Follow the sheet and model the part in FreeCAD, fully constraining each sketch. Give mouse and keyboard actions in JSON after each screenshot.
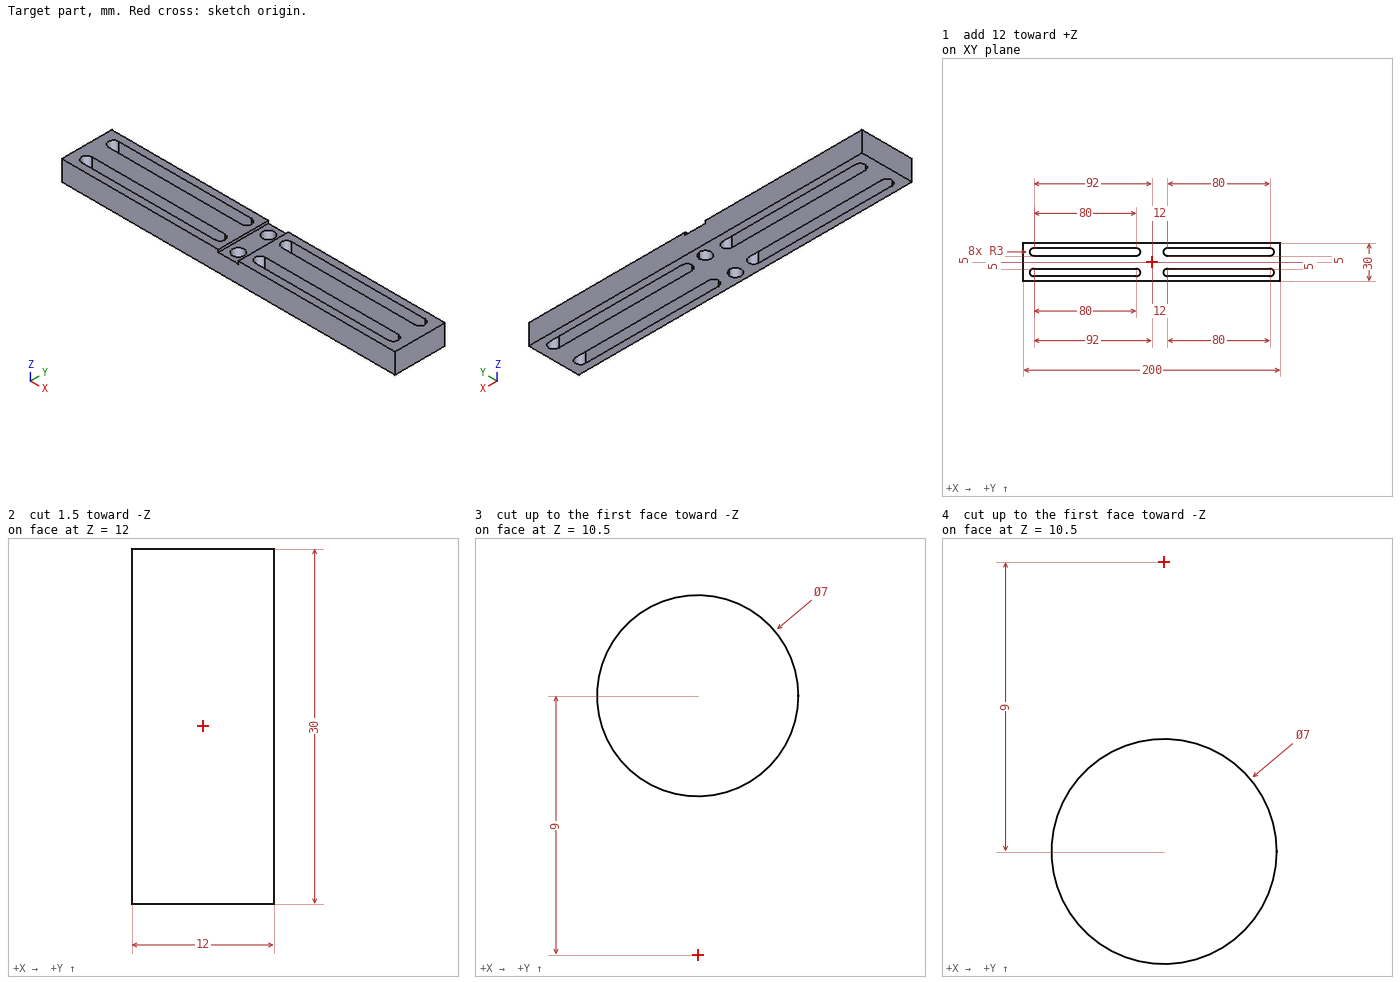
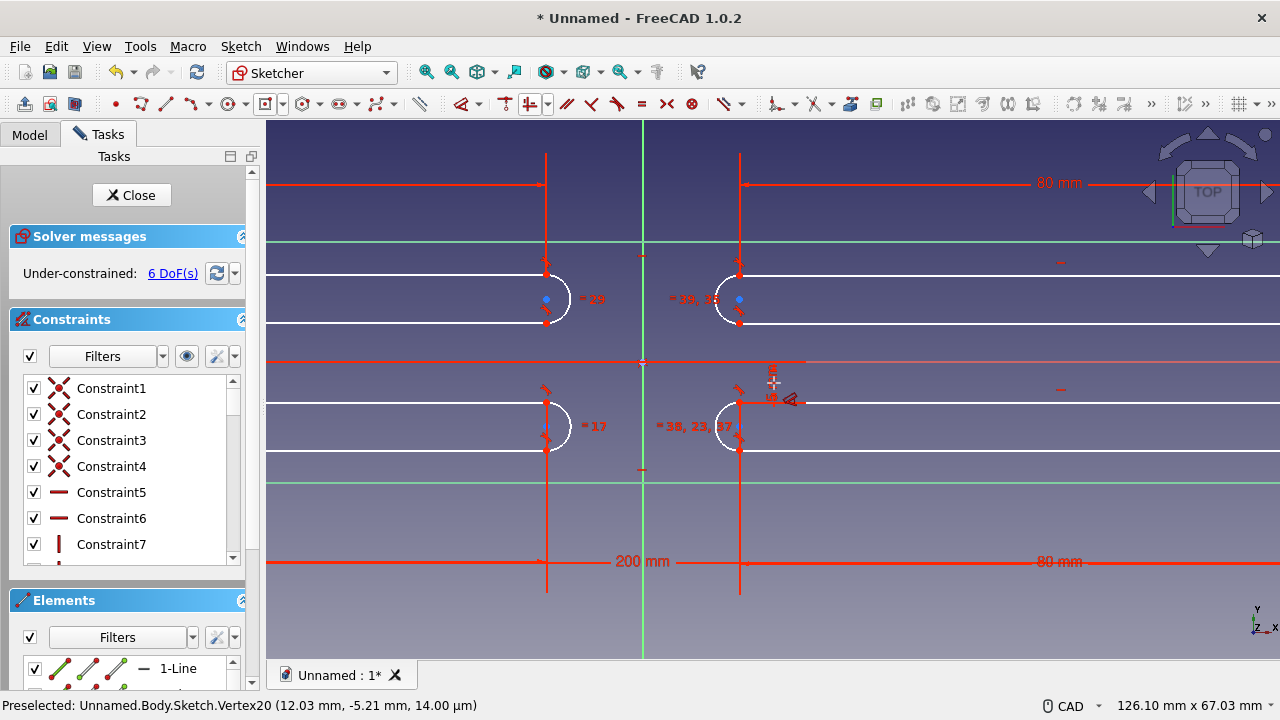
{"action": "scroll", "coordinate": [740, 405], "scroll_direction": "down", "scroll_amount": 5}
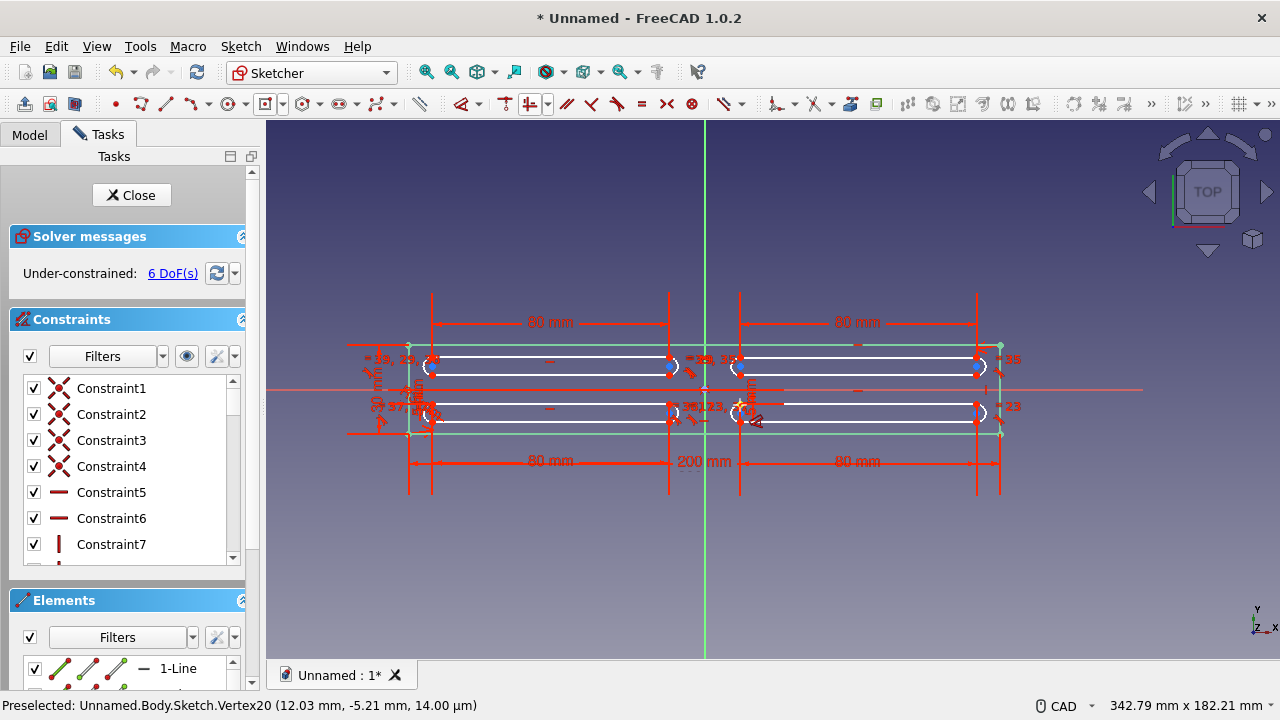
{"action": "scroll", "coordinate": [432, 375], "scroll_direction": "up", "scroll_amount": 5}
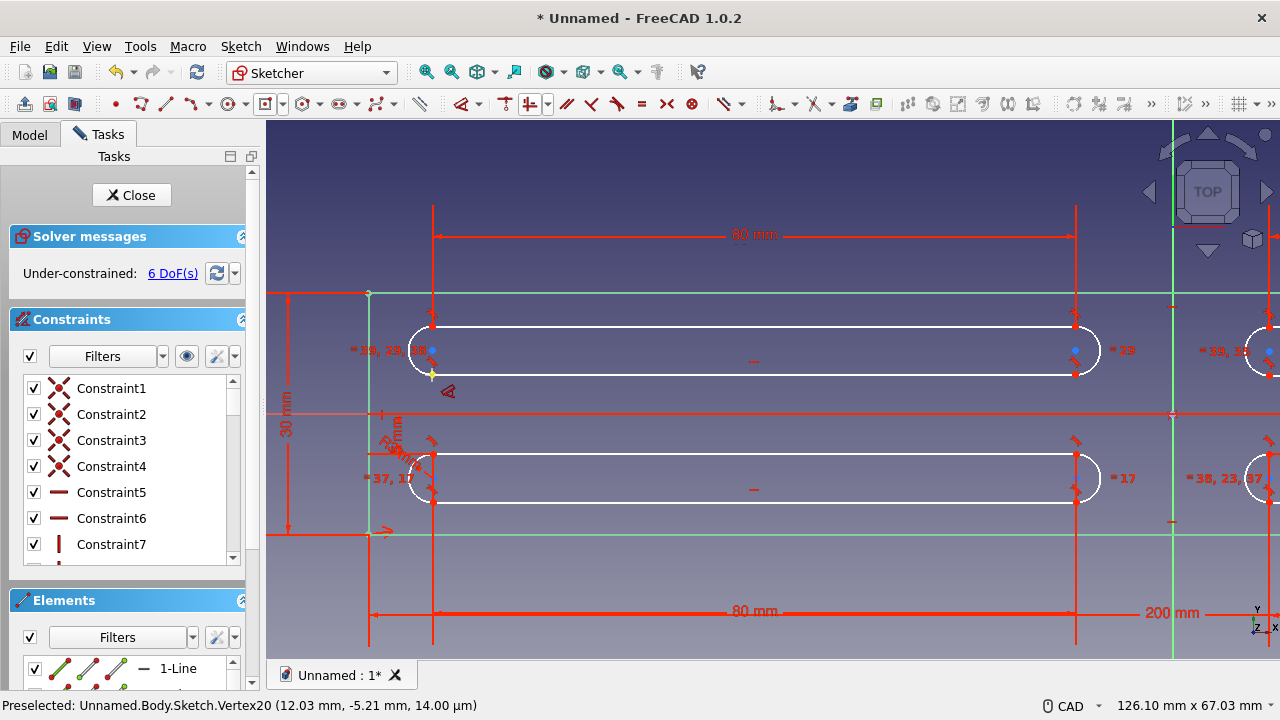
{"action": "left_click", "coordinate": [433, 375]}
{"action": "left_click", "coordinate": [399, 394]}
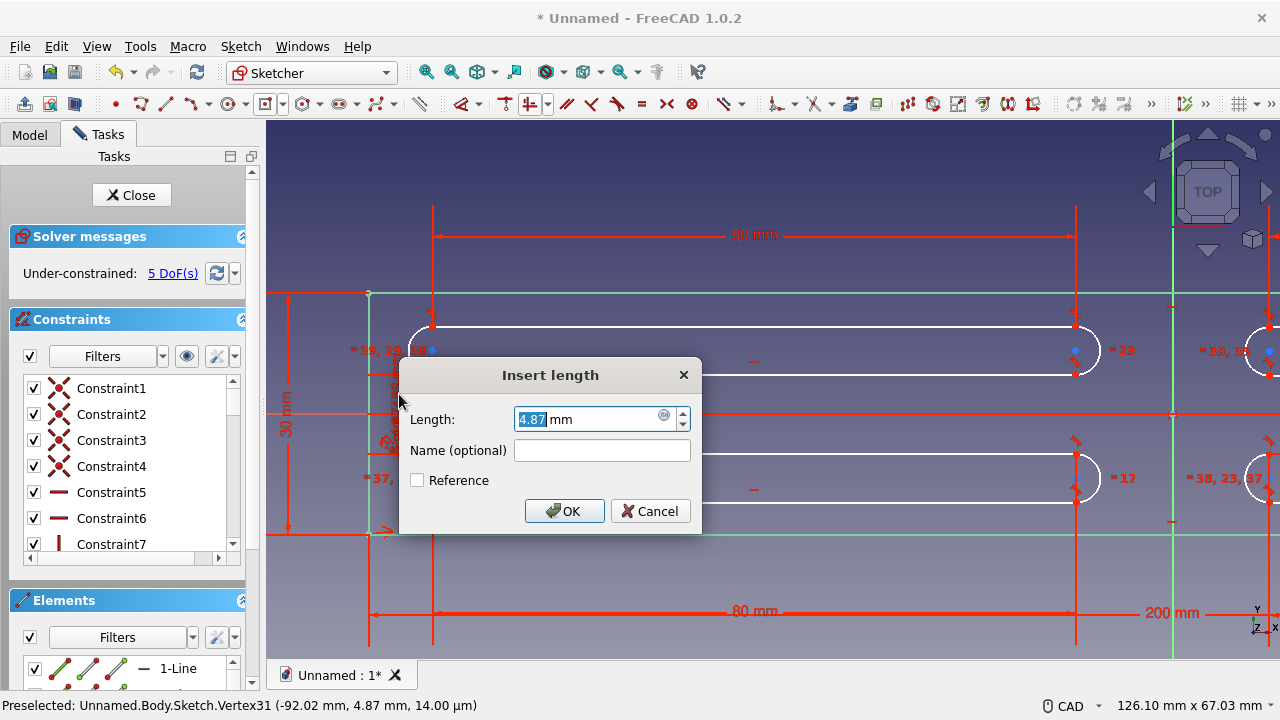
{"action": "type", "text": "5"}
{"action": "key", "text": "Return"}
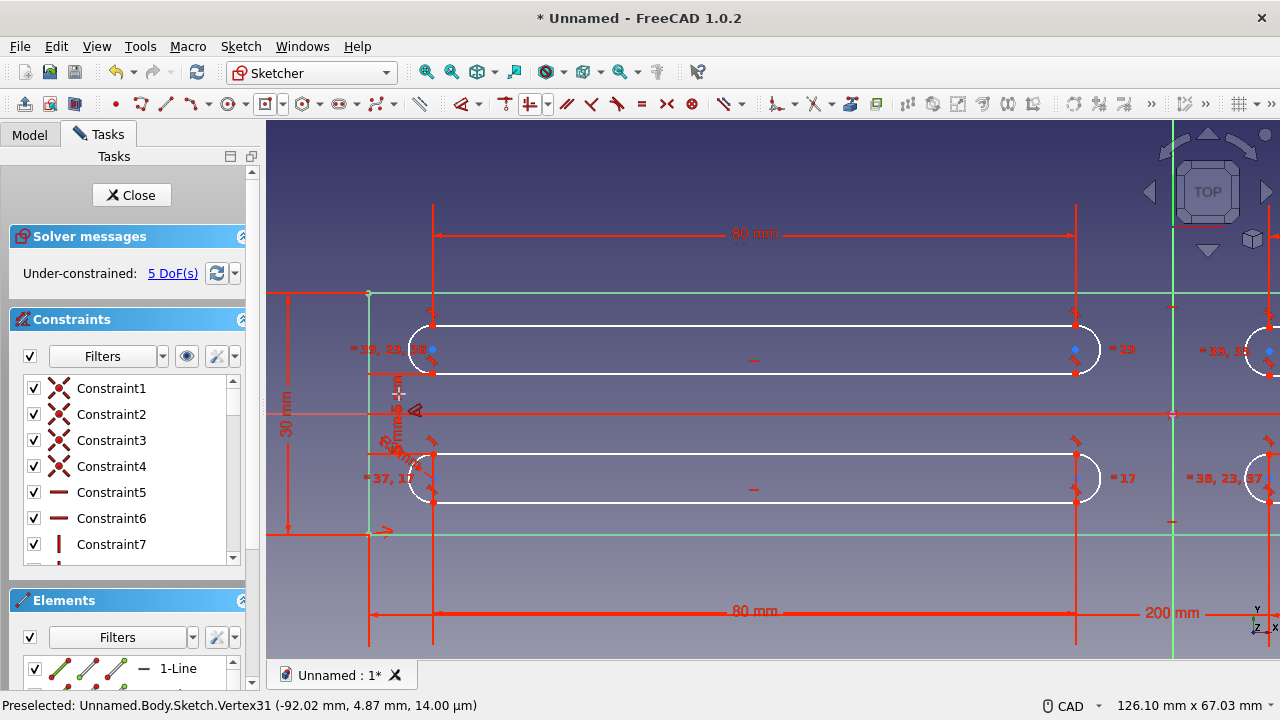
{"action": "scroll", "coordinate": [432, 375], "scroll_direction": "down", "scroll_amount": 5}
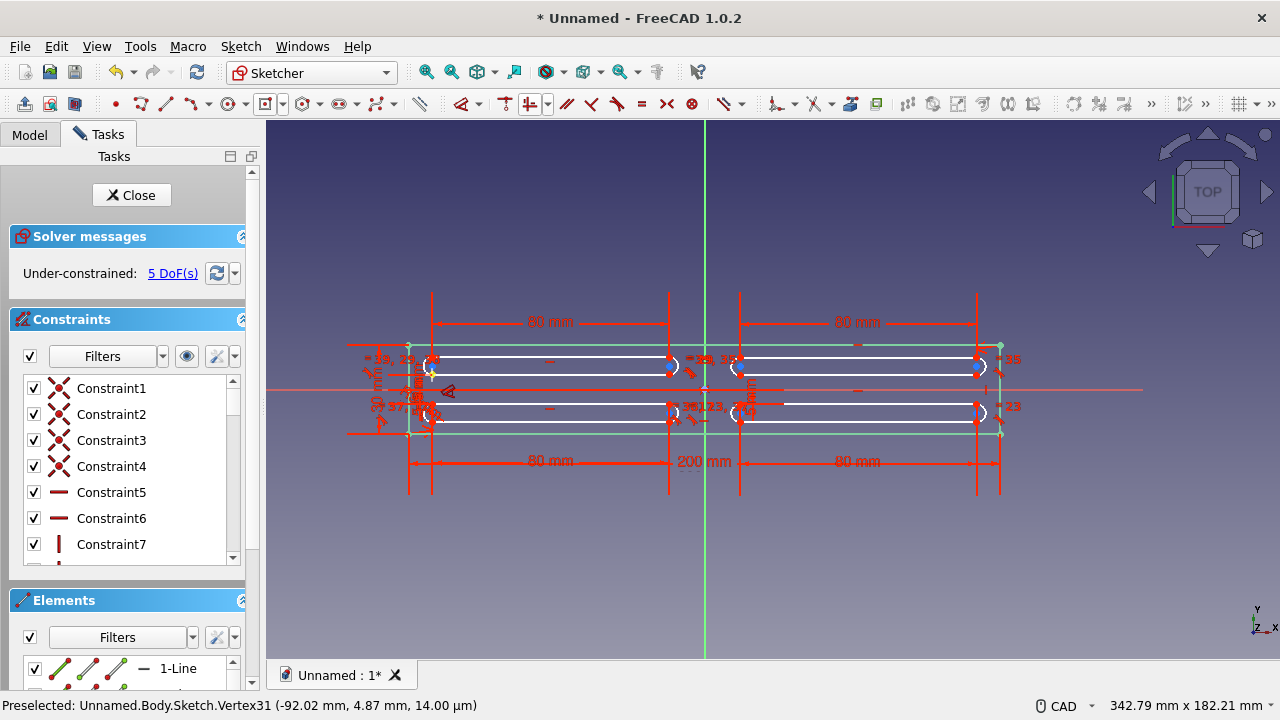
{"action": "scroll", "coordinate": [740, 375], "scroll_direction": "up", "scroll_amount": 5}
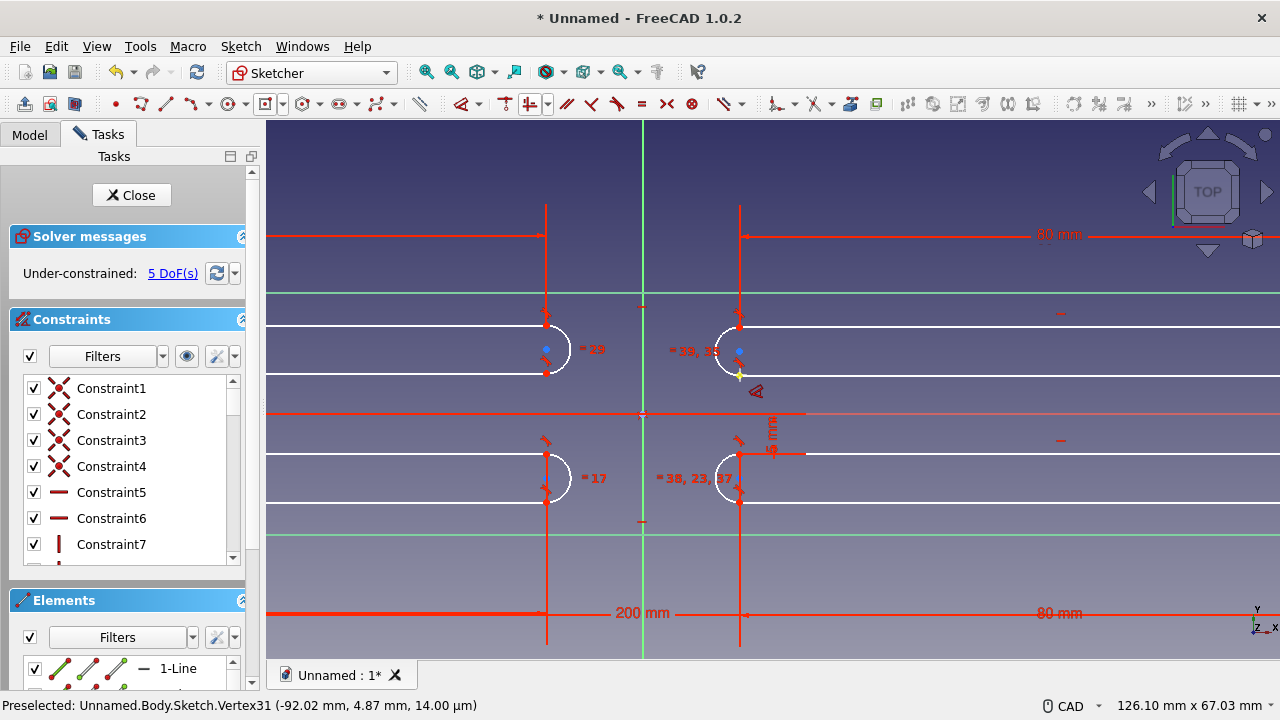
{"action": "left_click", "coordinate": [740, 376]}
{"action": "left_click", "coordinate": [774, 395]}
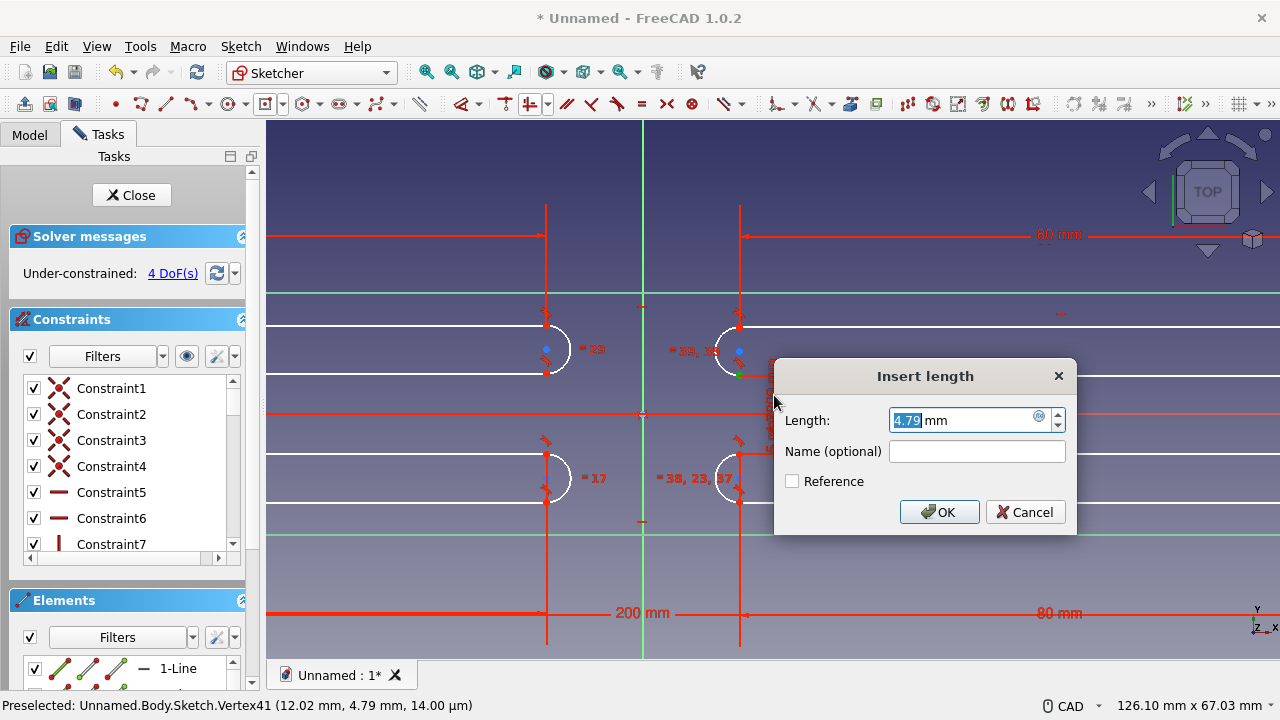
{"action": "type", "text": "5"}
{"action": "key", "text": "Return"}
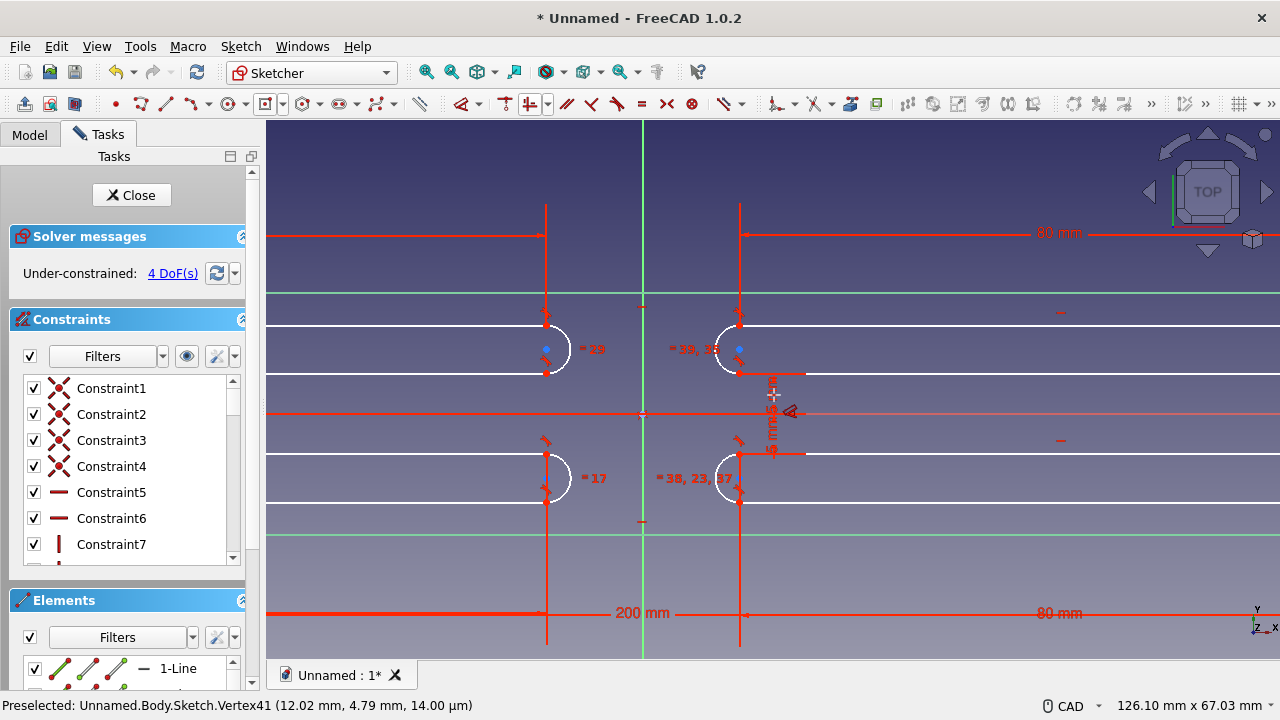
{"action": "scroll", "coordinate": [740, 375], "scroll_direction": "down", "scroll_amount": 5}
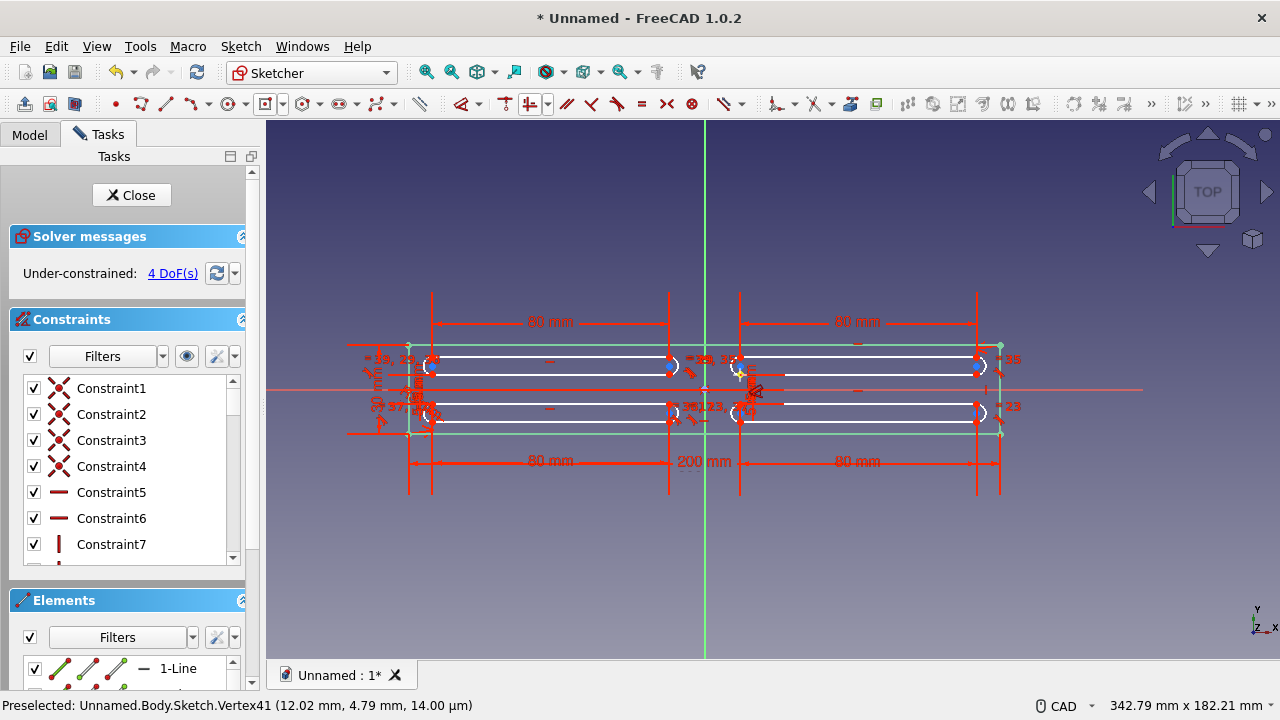
{"action": "scroll", "coordinate": [432, 404], "scroll_direction": "up", "scroll_amount": 2}